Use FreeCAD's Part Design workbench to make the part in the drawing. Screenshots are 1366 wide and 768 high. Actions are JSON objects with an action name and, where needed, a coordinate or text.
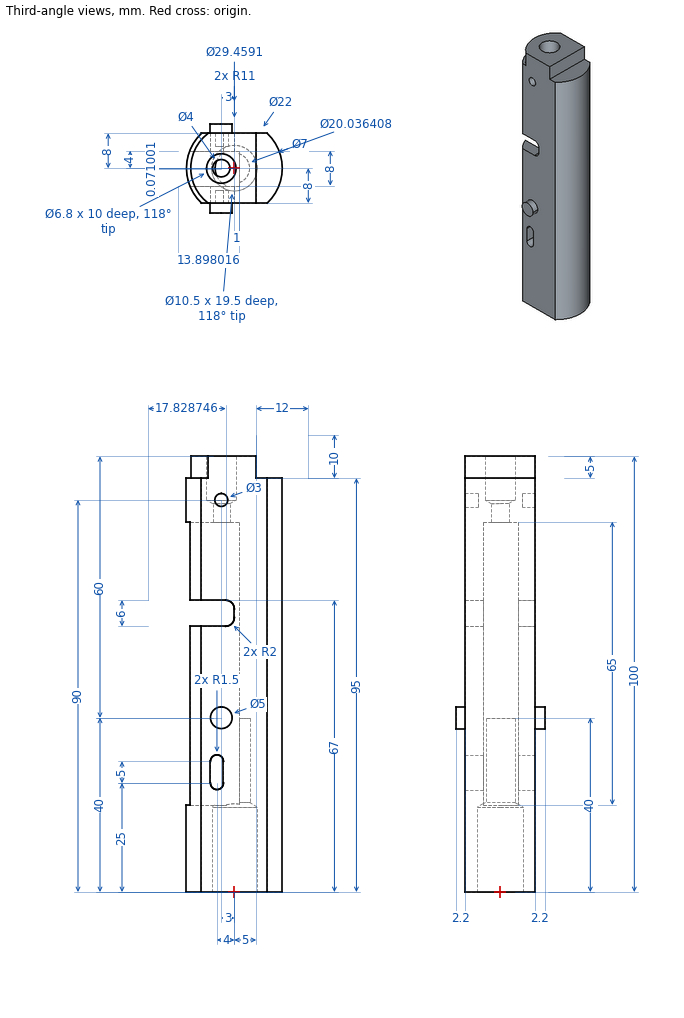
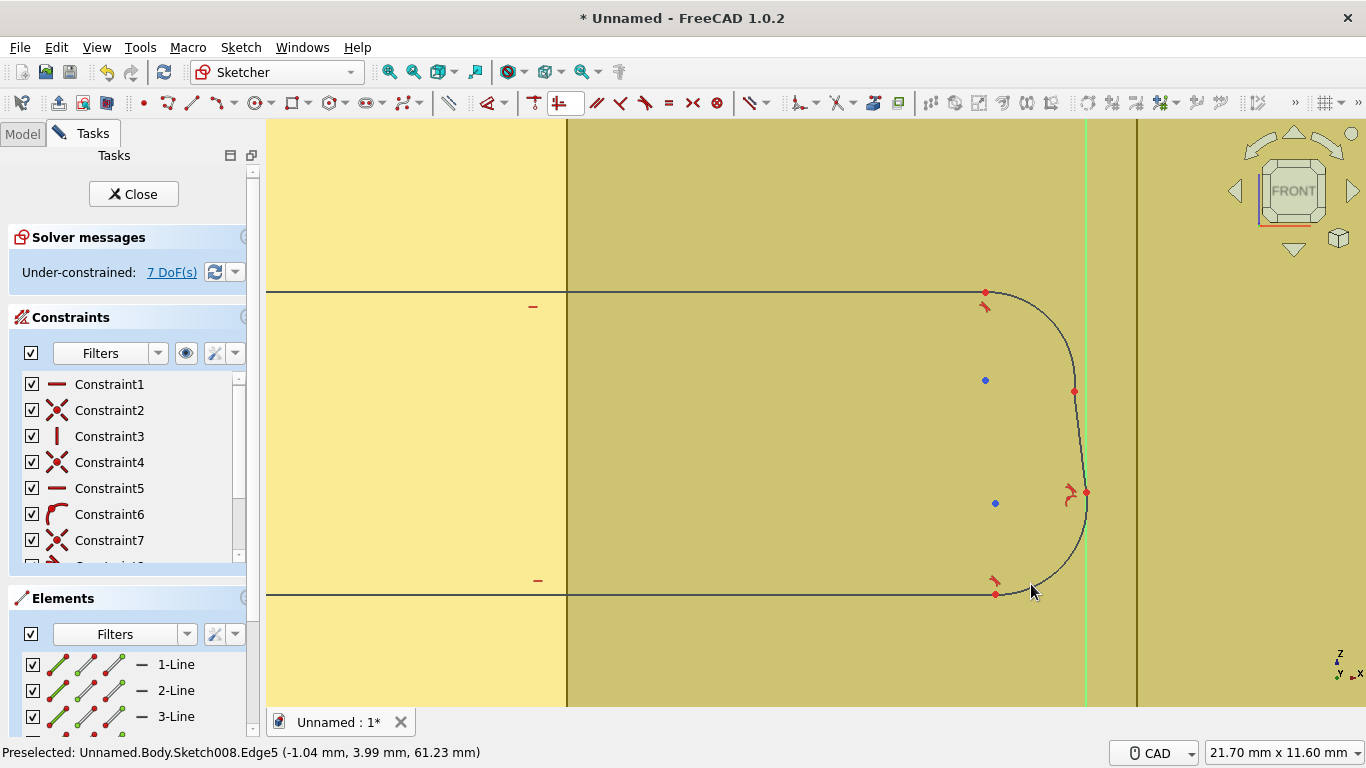
{"action": "left_click", "coordinate": [1083, 462]}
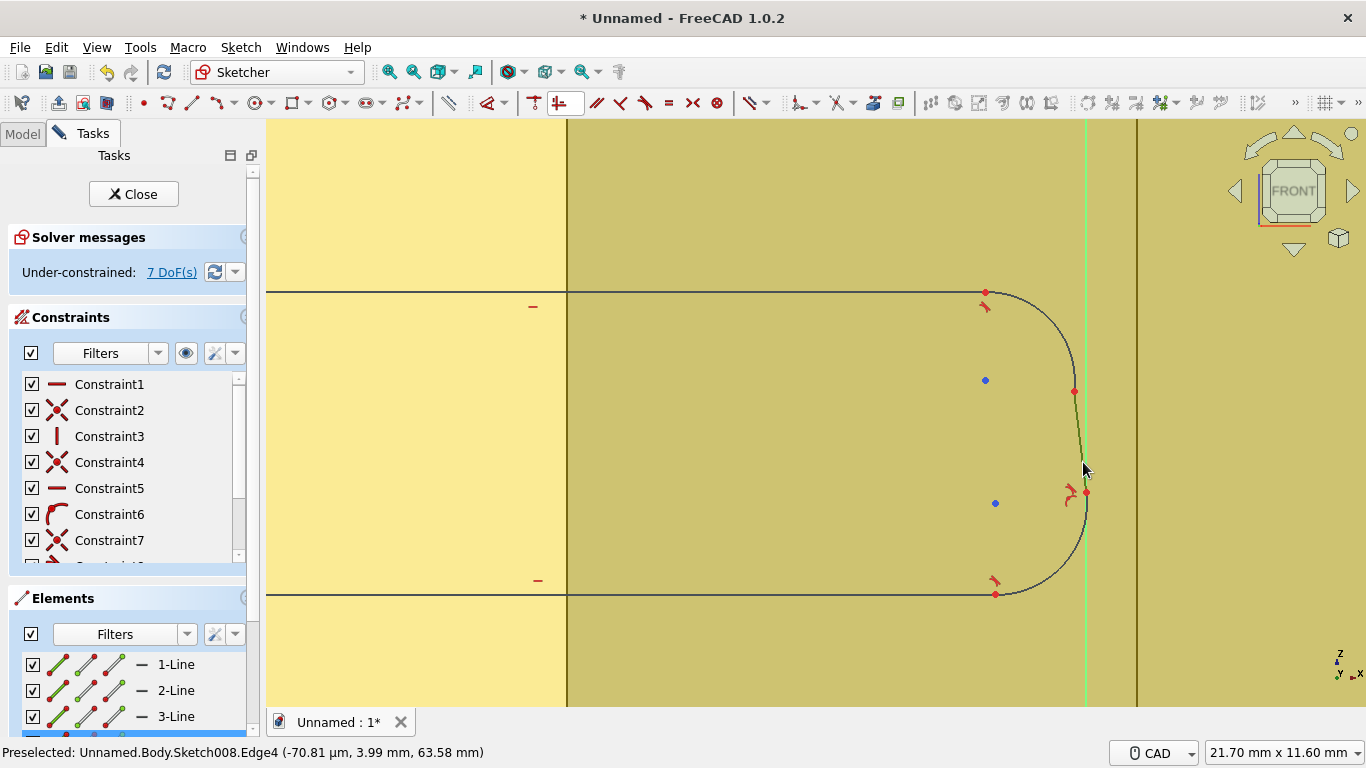
{"action": "left_click", "coordinate": [1068, 348]}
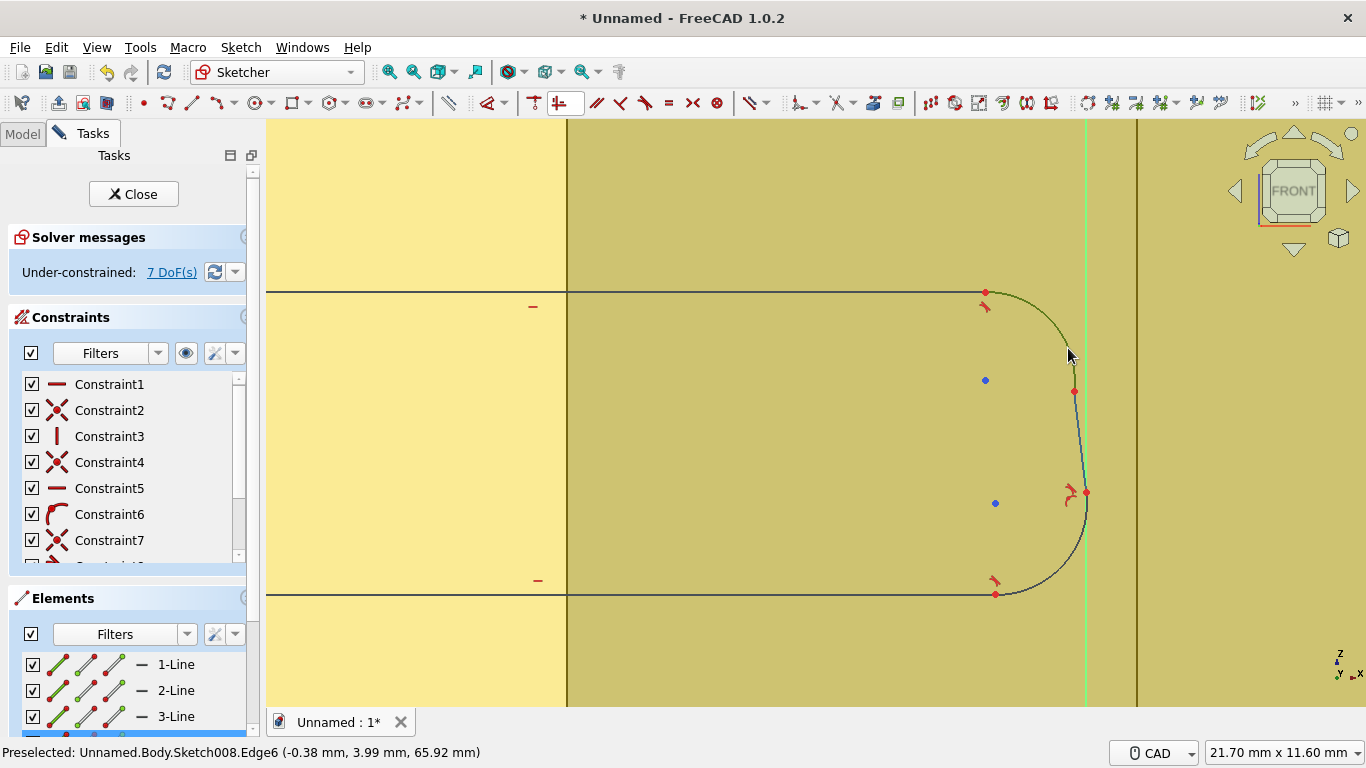
{"action": "key", "text": "t"}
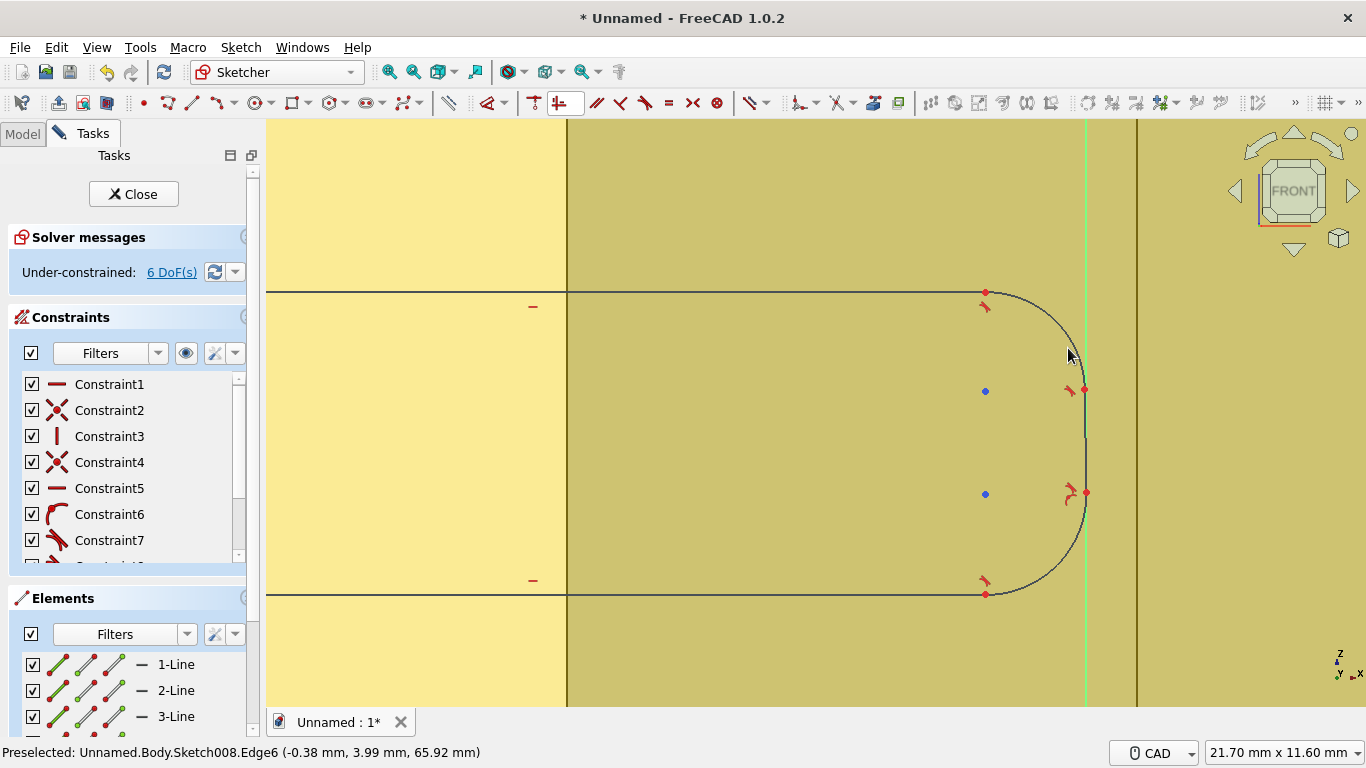
{"action": "left_click", "coordinate": [1086, 462]}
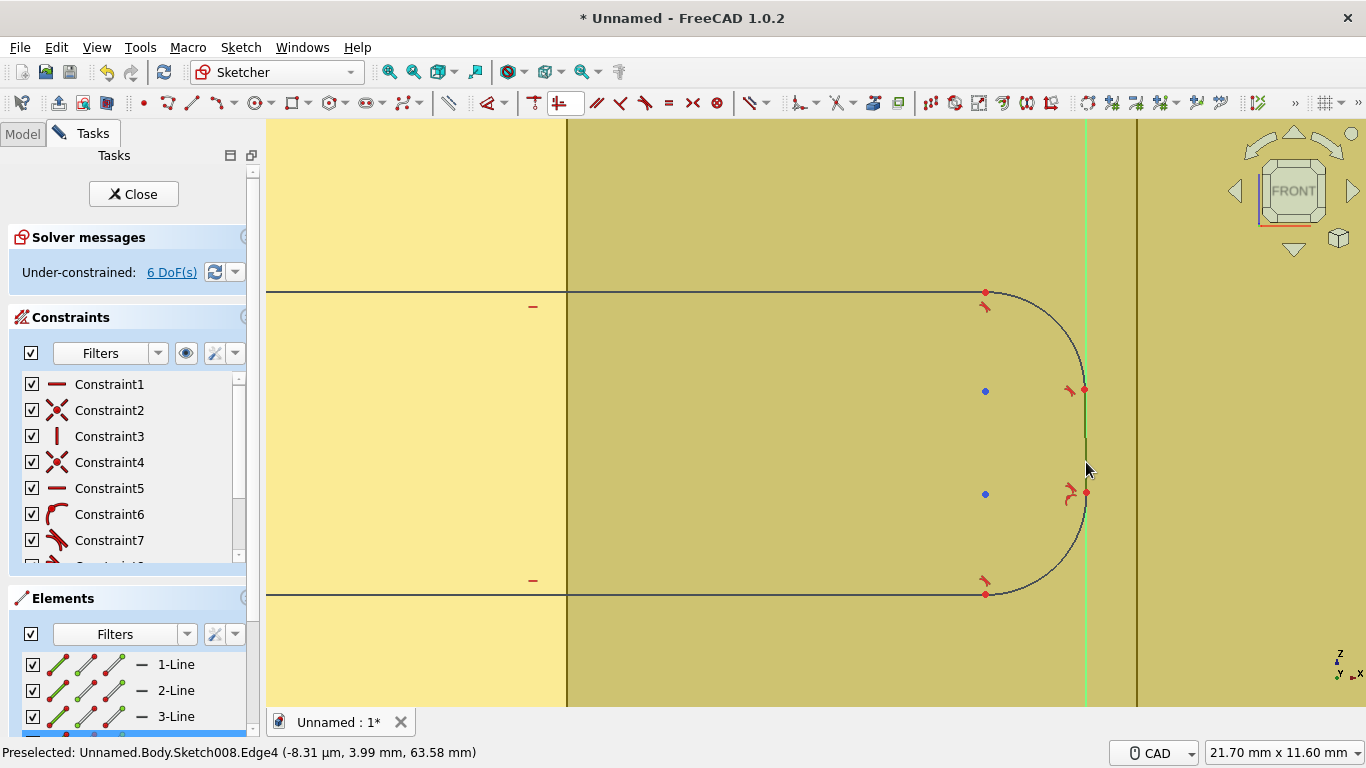
{"action": "key", "text": "v"}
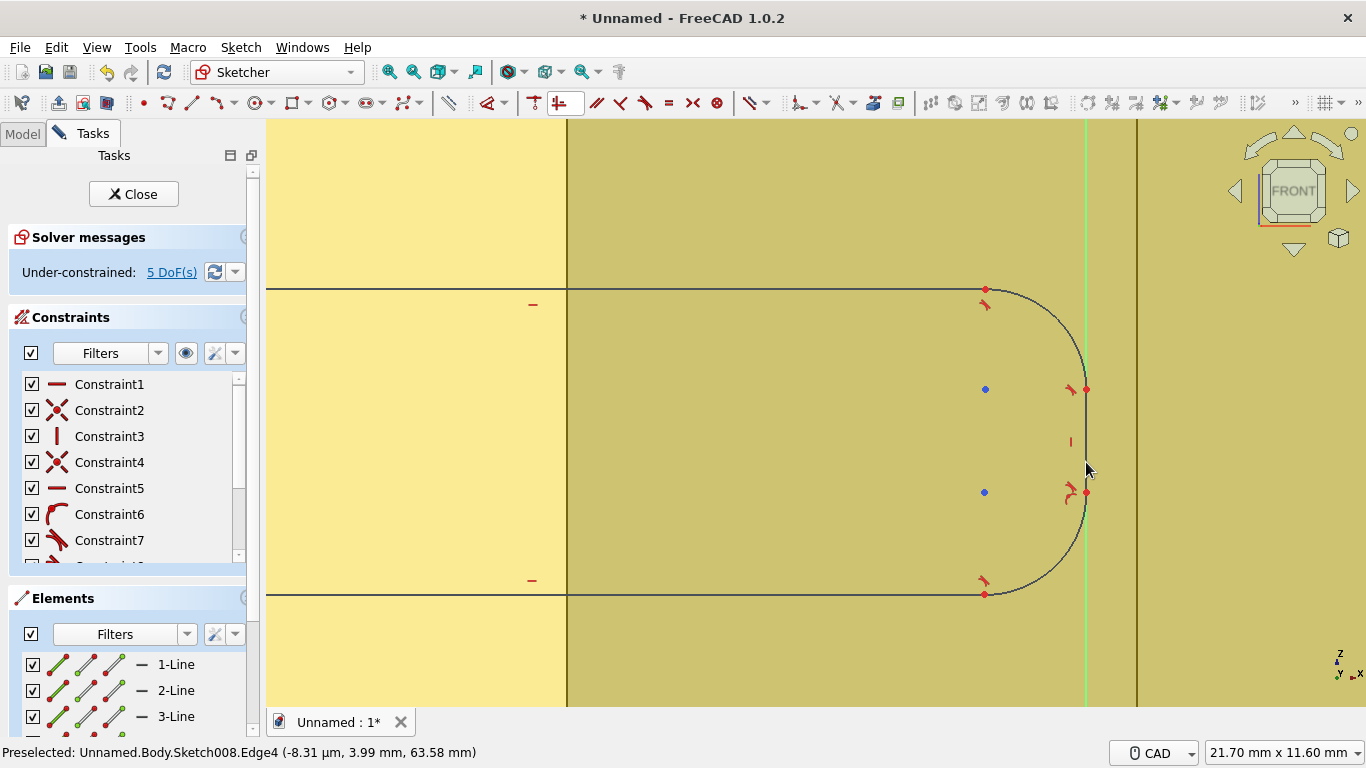
{"action": "left_click", "coordinate": [1031, 584]}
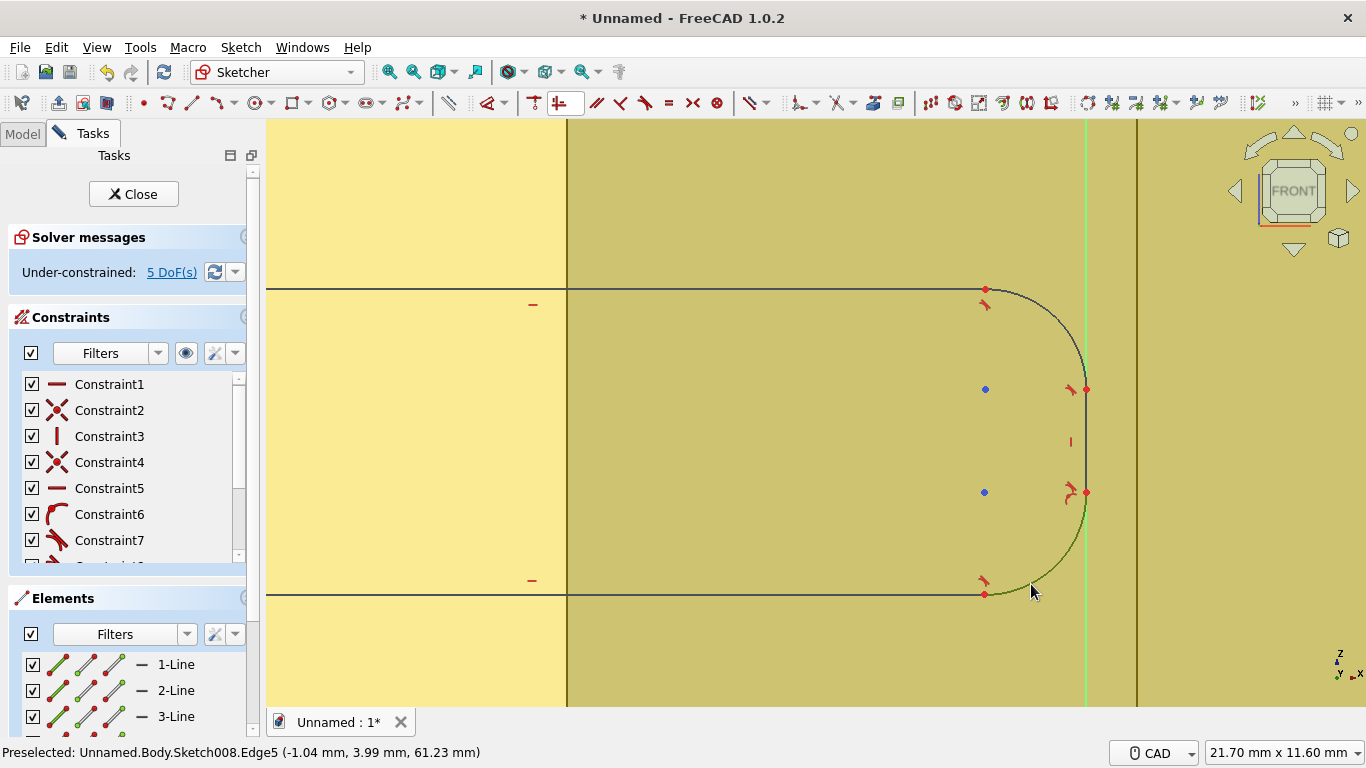
{"action": "scroll", "coordinate": [1075, 344], "scroll_direction": "up", "scroll_amount": 2}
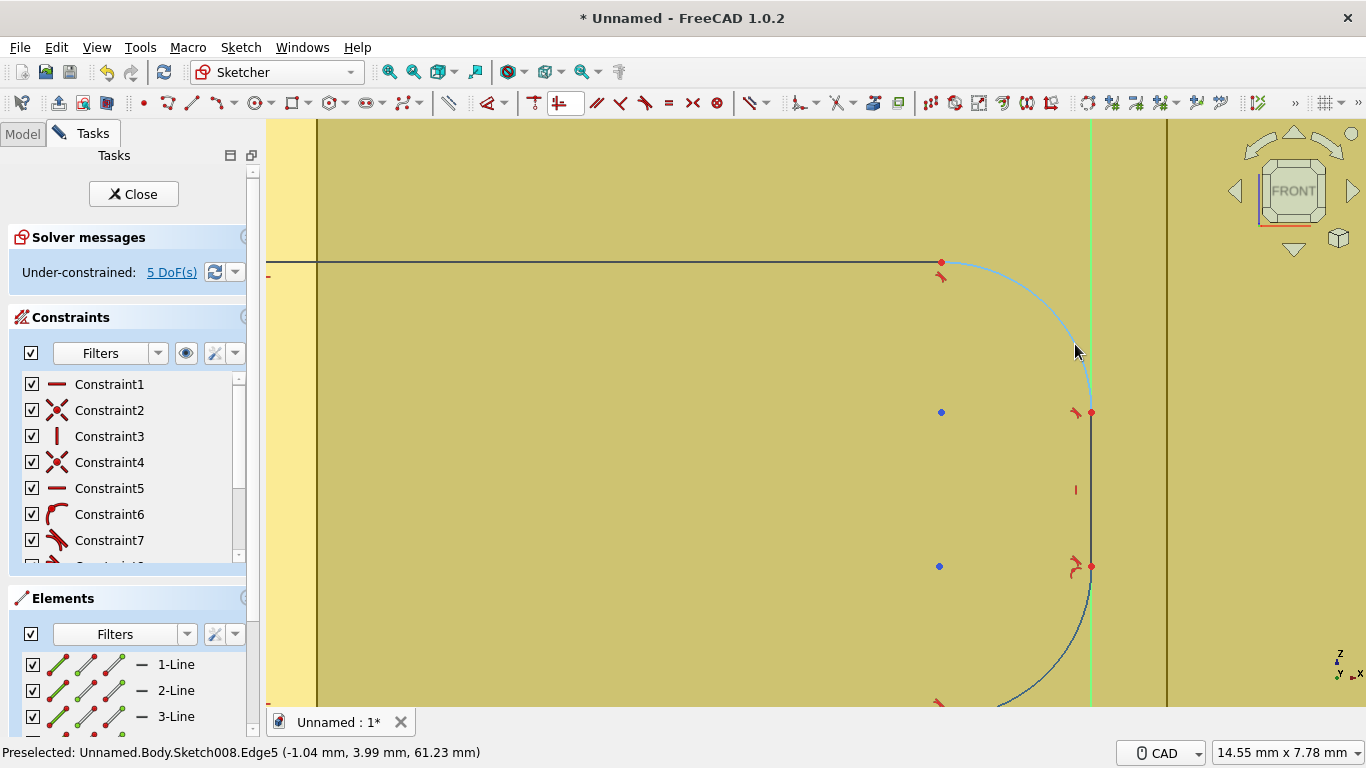
{"action": "left_click", "coordinate": [1075, 344]}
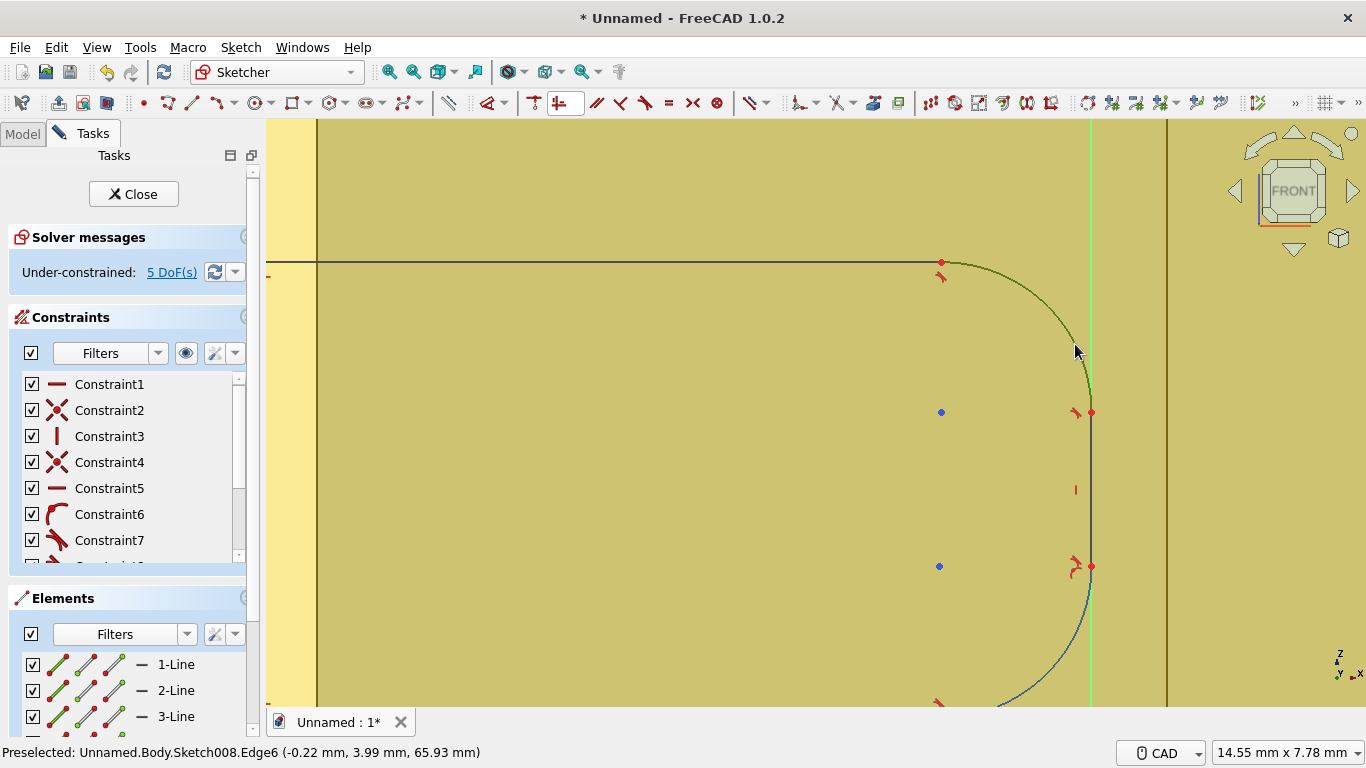
{"action": "key", "text": "e"}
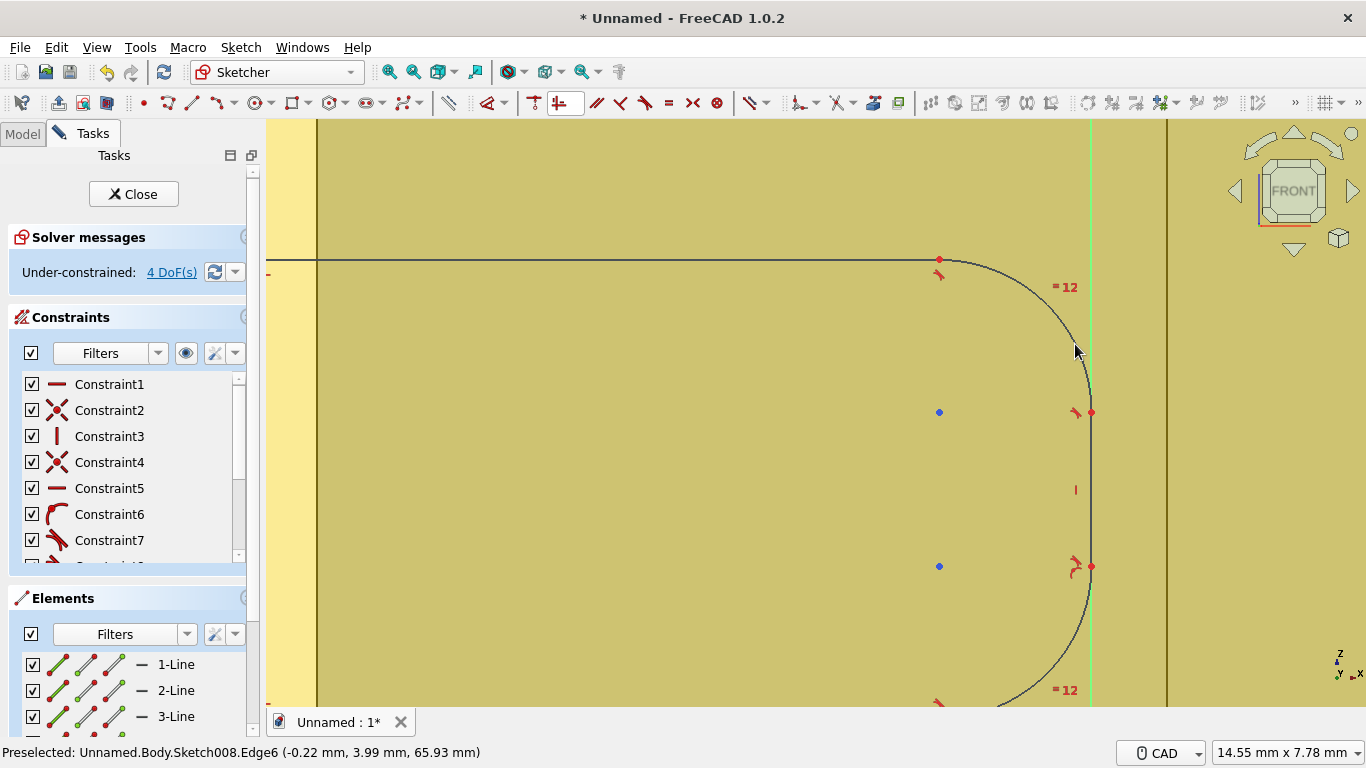
{"action": "left_click", "coordinate": [488, 104]}